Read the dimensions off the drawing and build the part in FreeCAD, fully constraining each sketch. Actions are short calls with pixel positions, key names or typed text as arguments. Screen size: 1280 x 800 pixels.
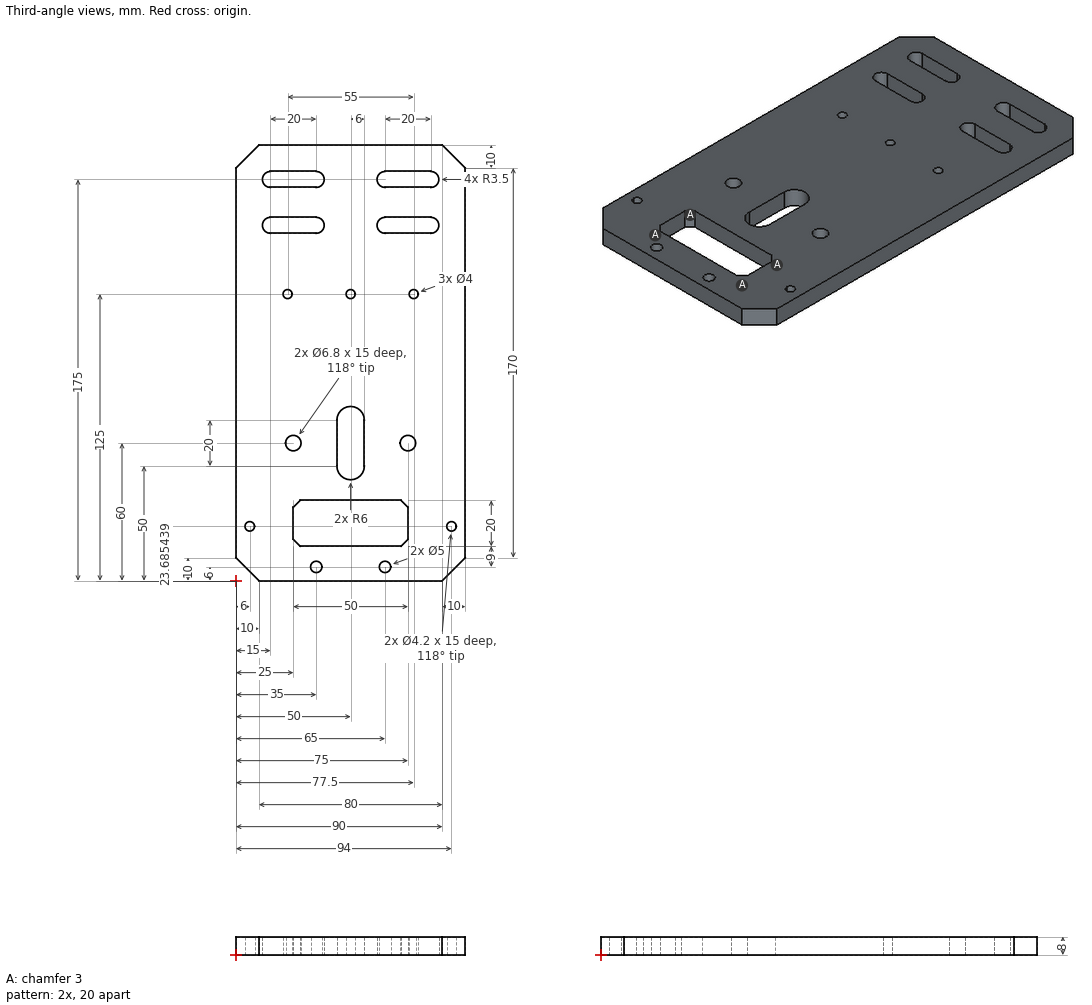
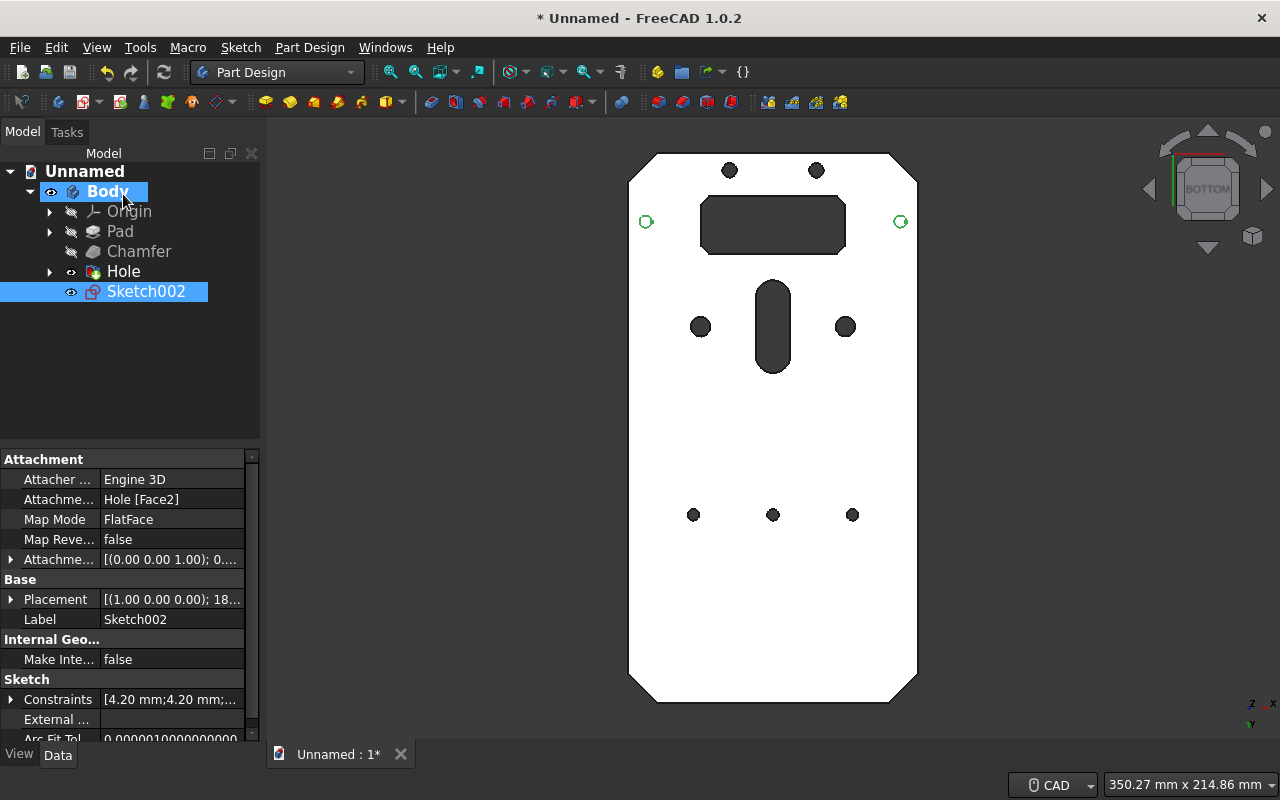
click(456, 102)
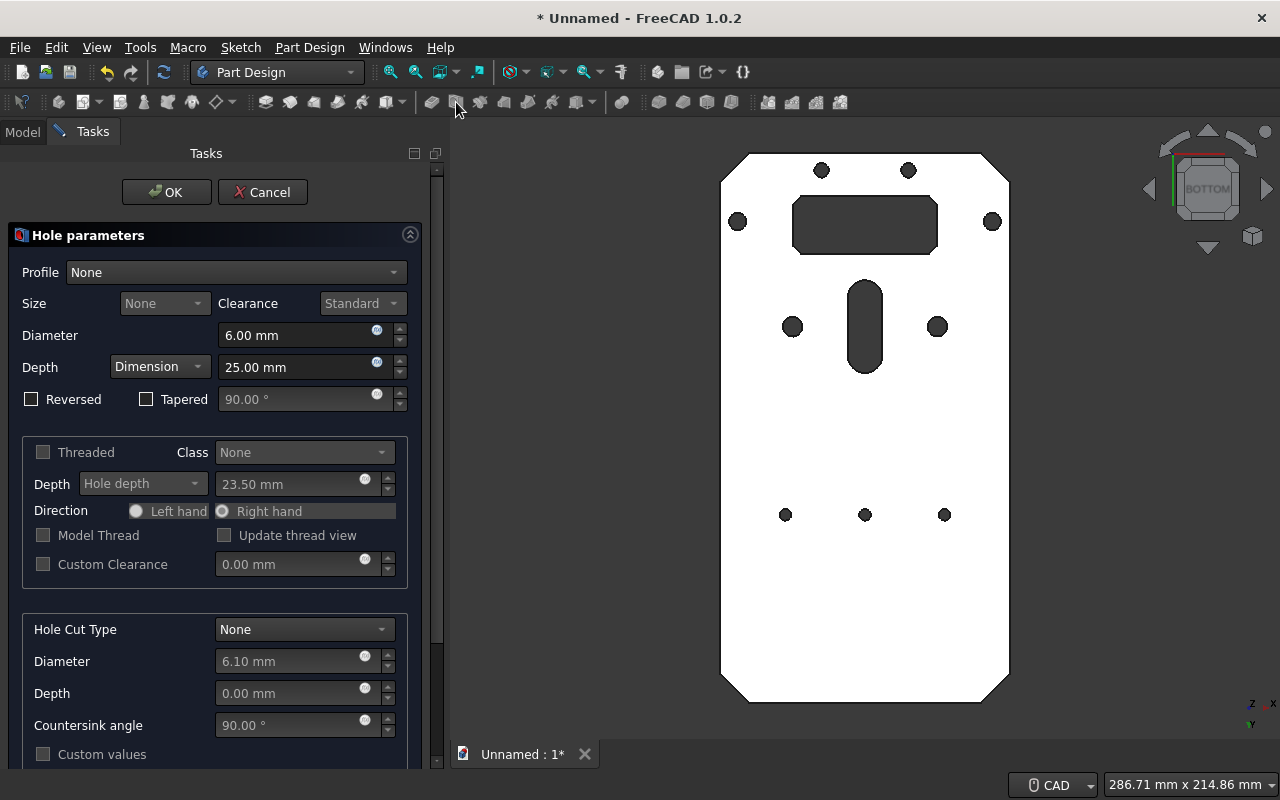
triple_click(305, 335)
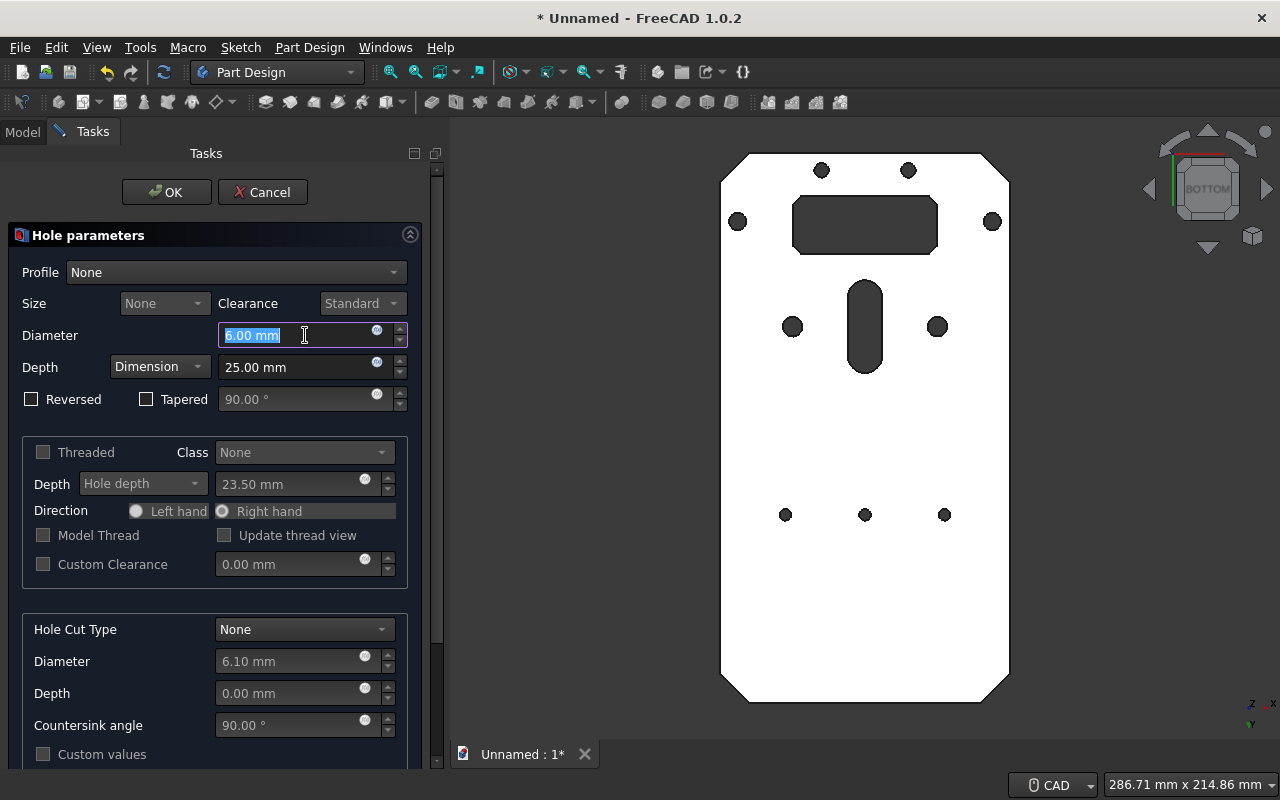
text(4.2)
key(Tab)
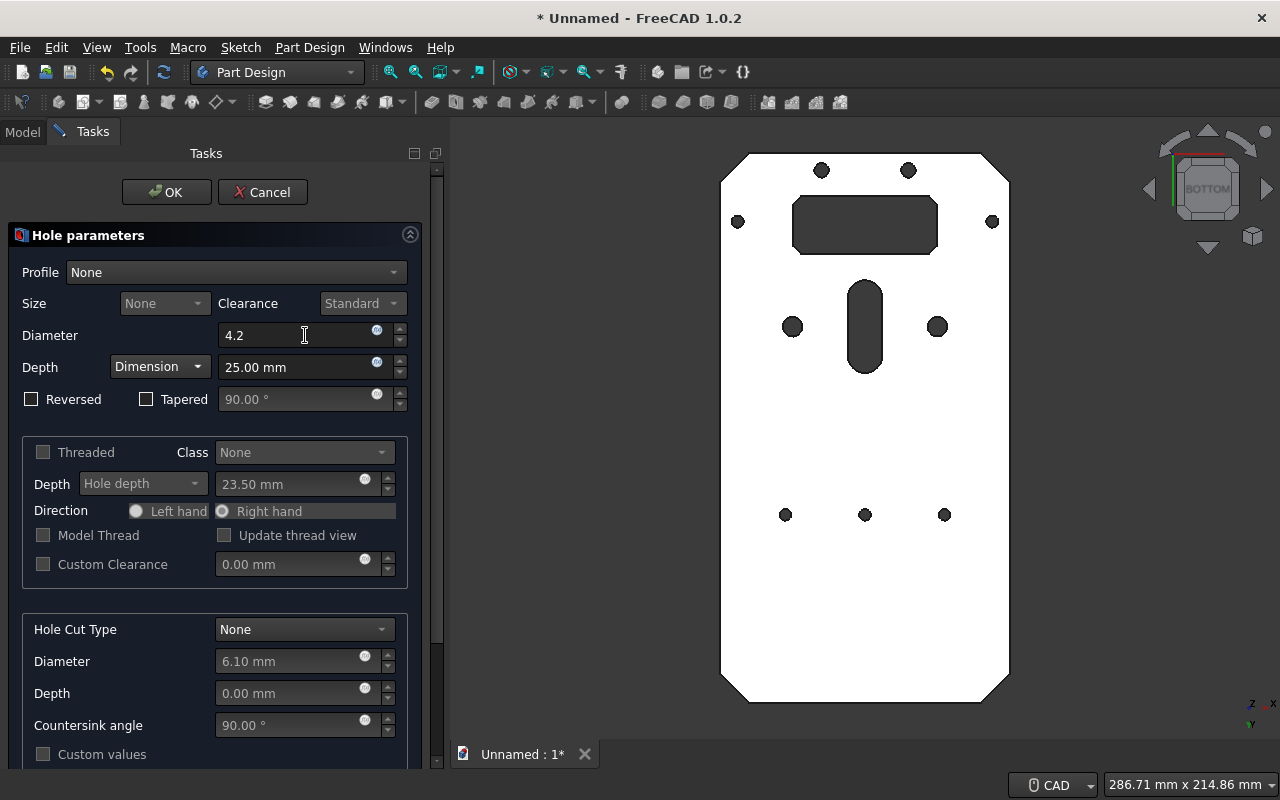
triple_click(305, 367)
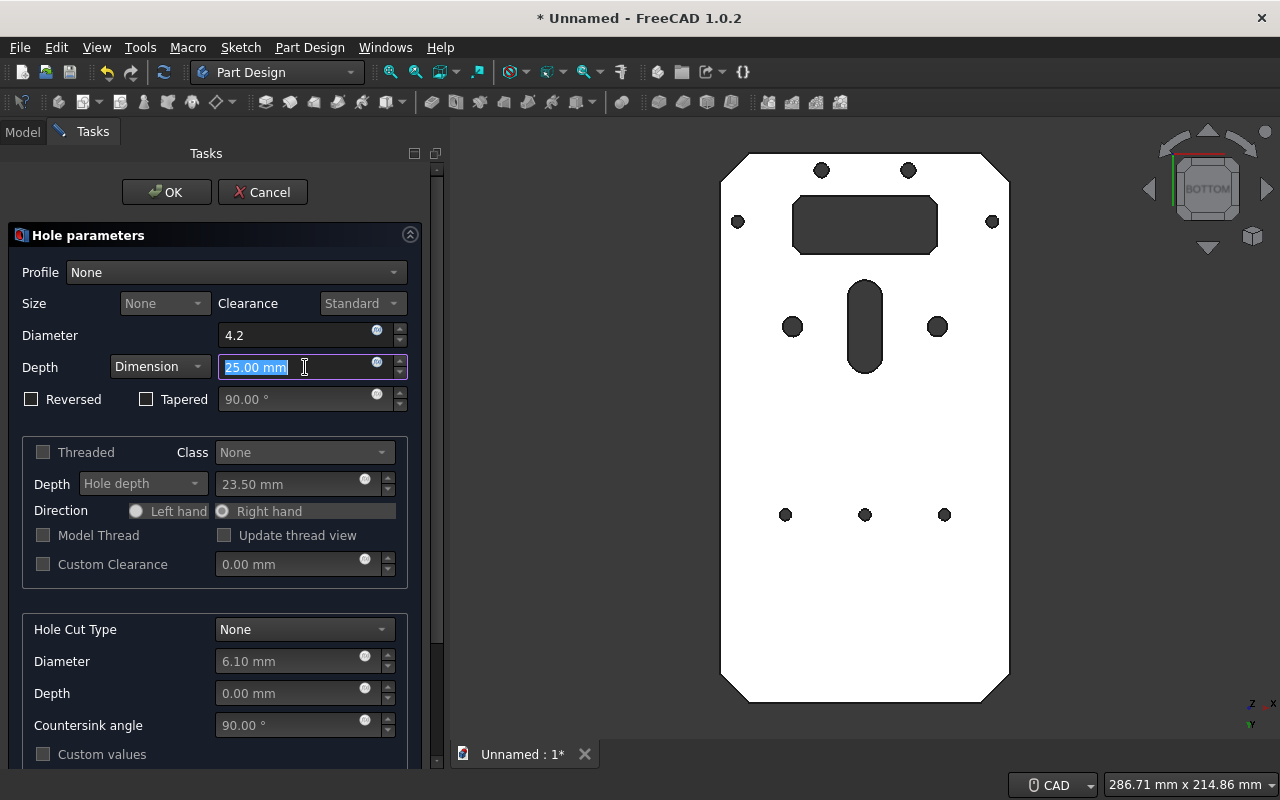
text(15)
key(Tab)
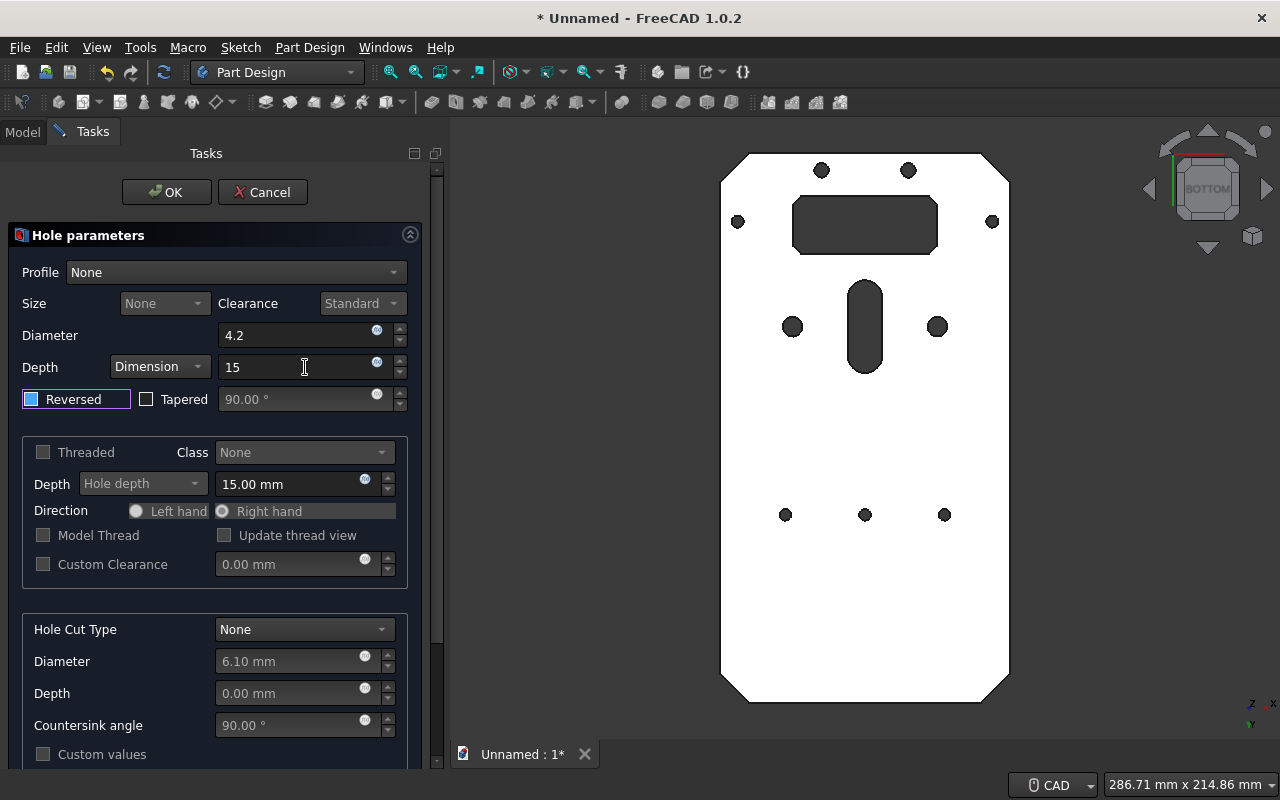
click(167, 192)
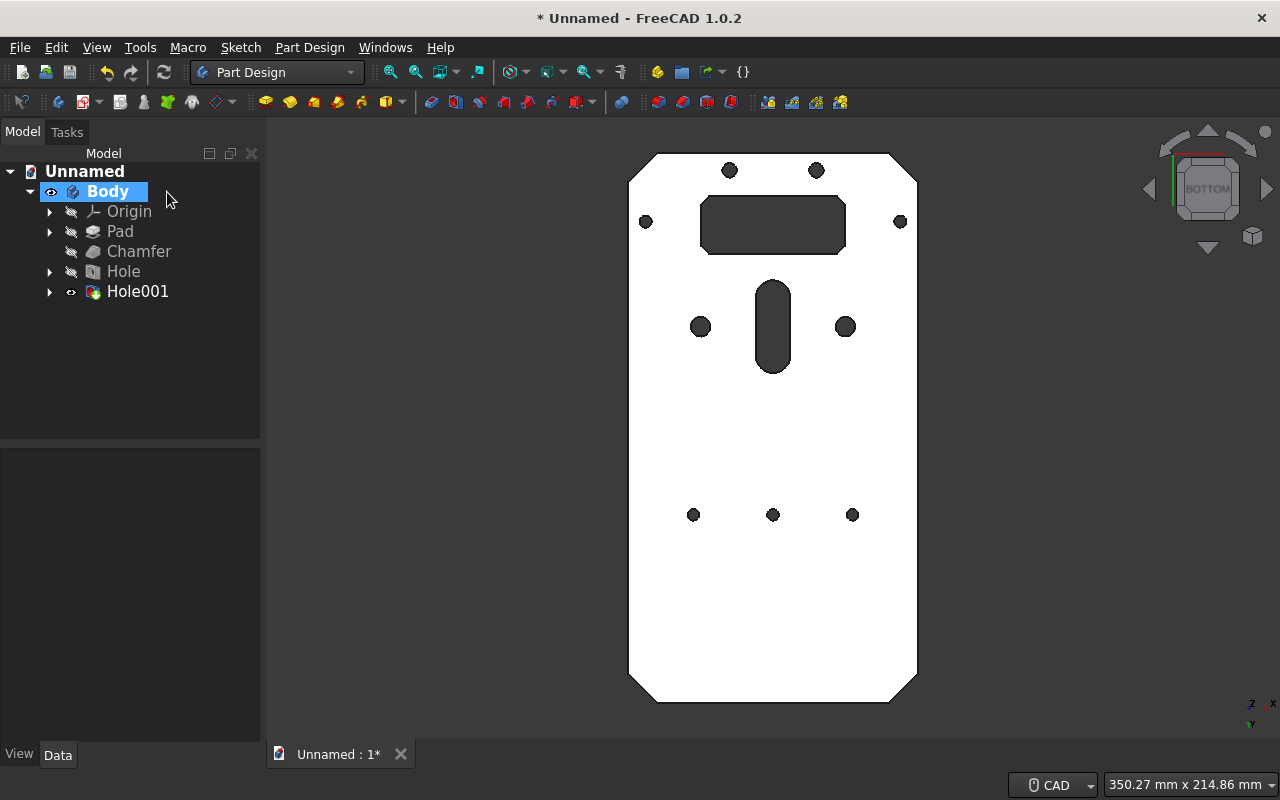
click(84, 102)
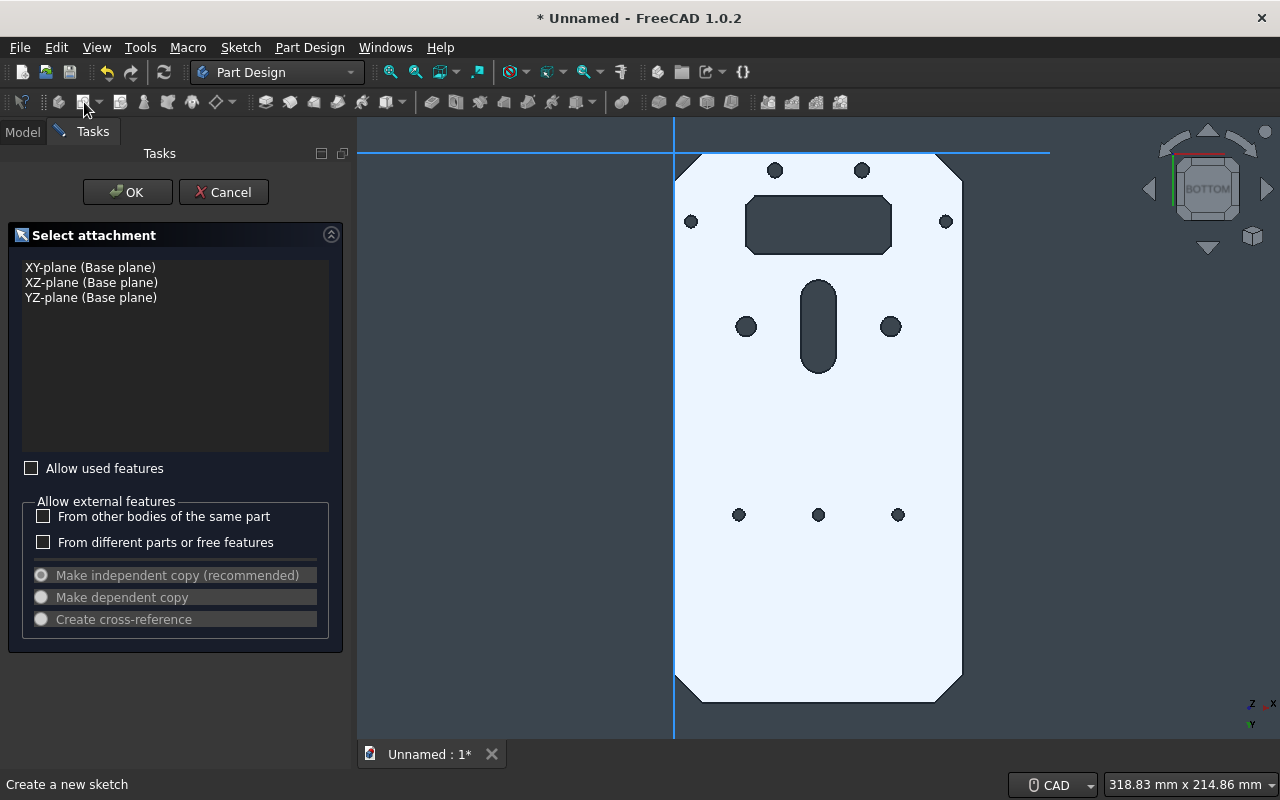
click(82, 268)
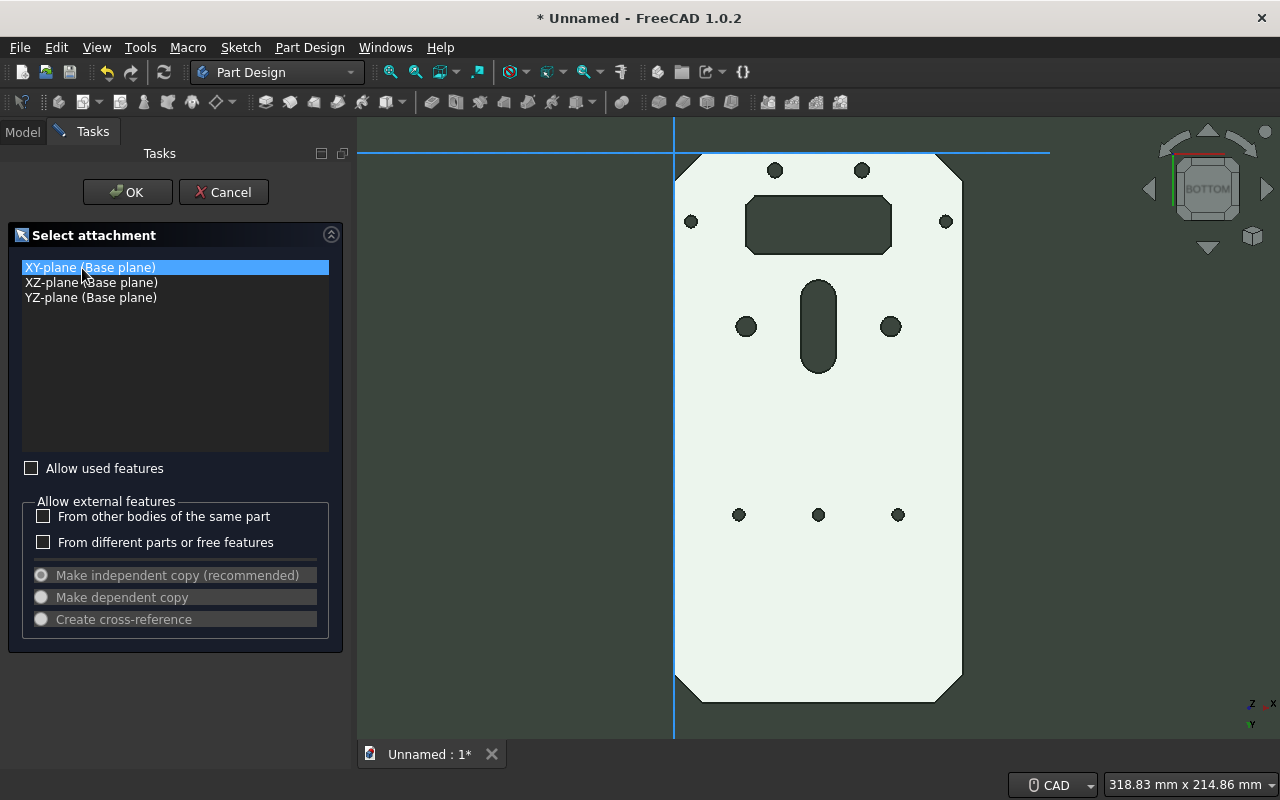
click(128, 192)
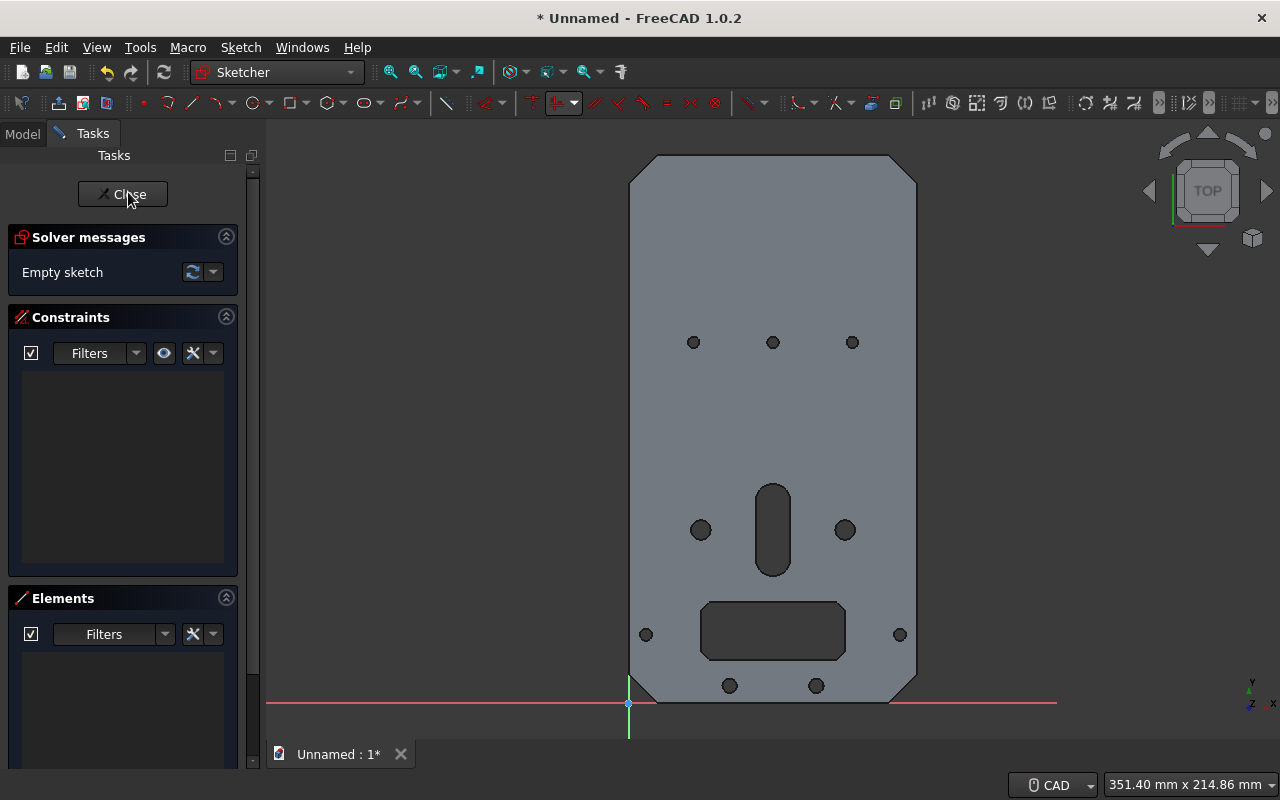
key(q)
key(s)